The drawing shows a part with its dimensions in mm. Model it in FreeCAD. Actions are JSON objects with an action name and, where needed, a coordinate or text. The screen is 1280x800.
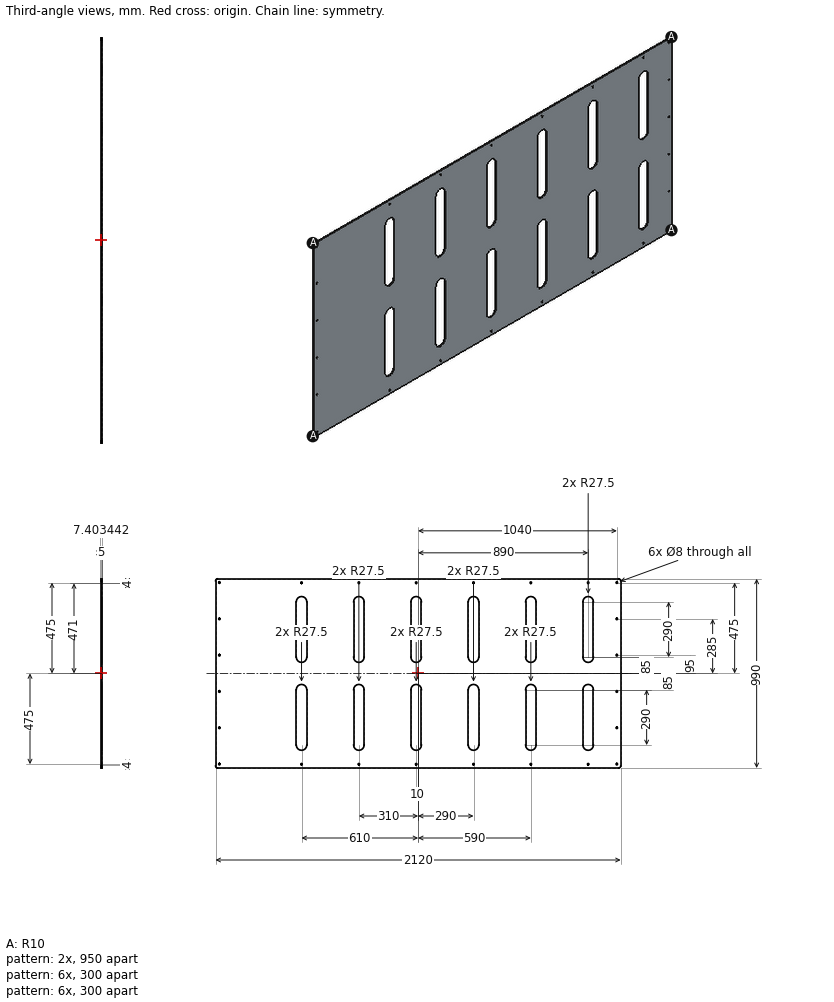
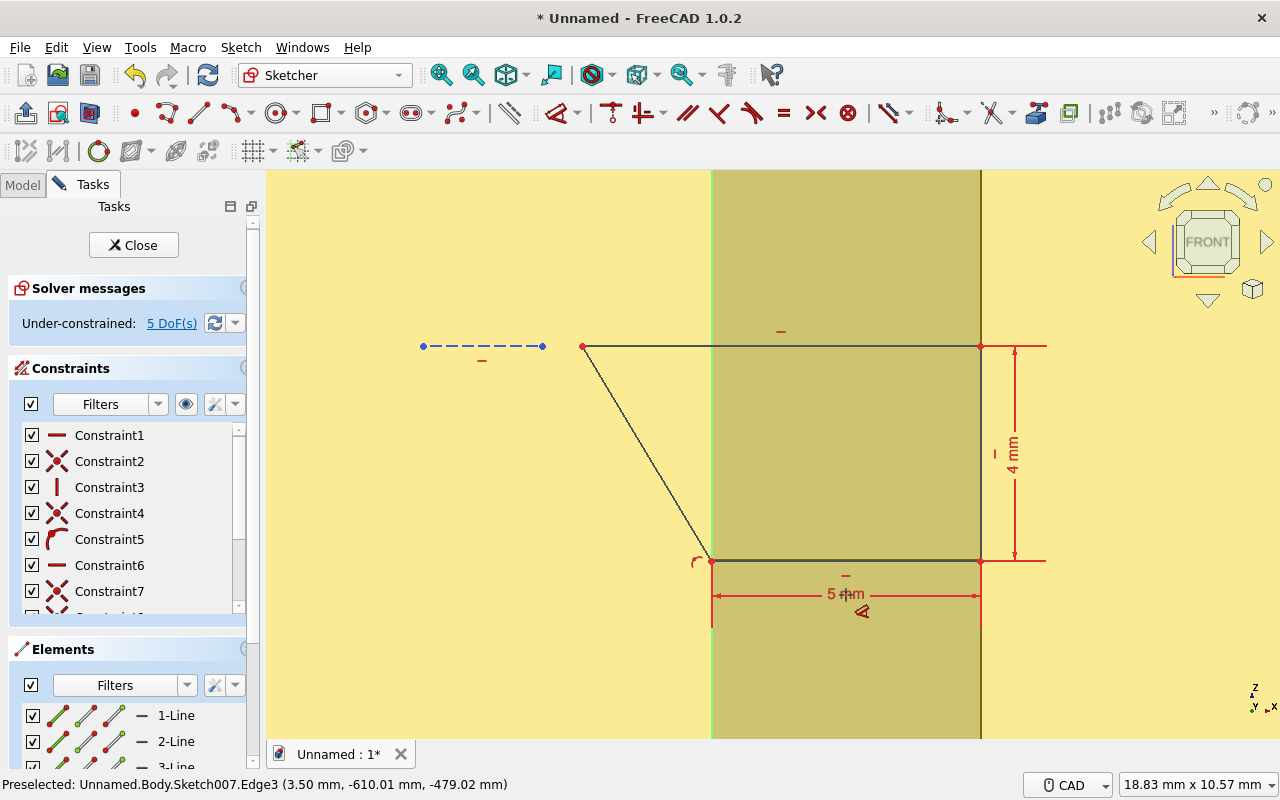
{"action": "left_click", "coordinate": [582, 346]}
{"action": "left_click", "coordinate": [548, 272]}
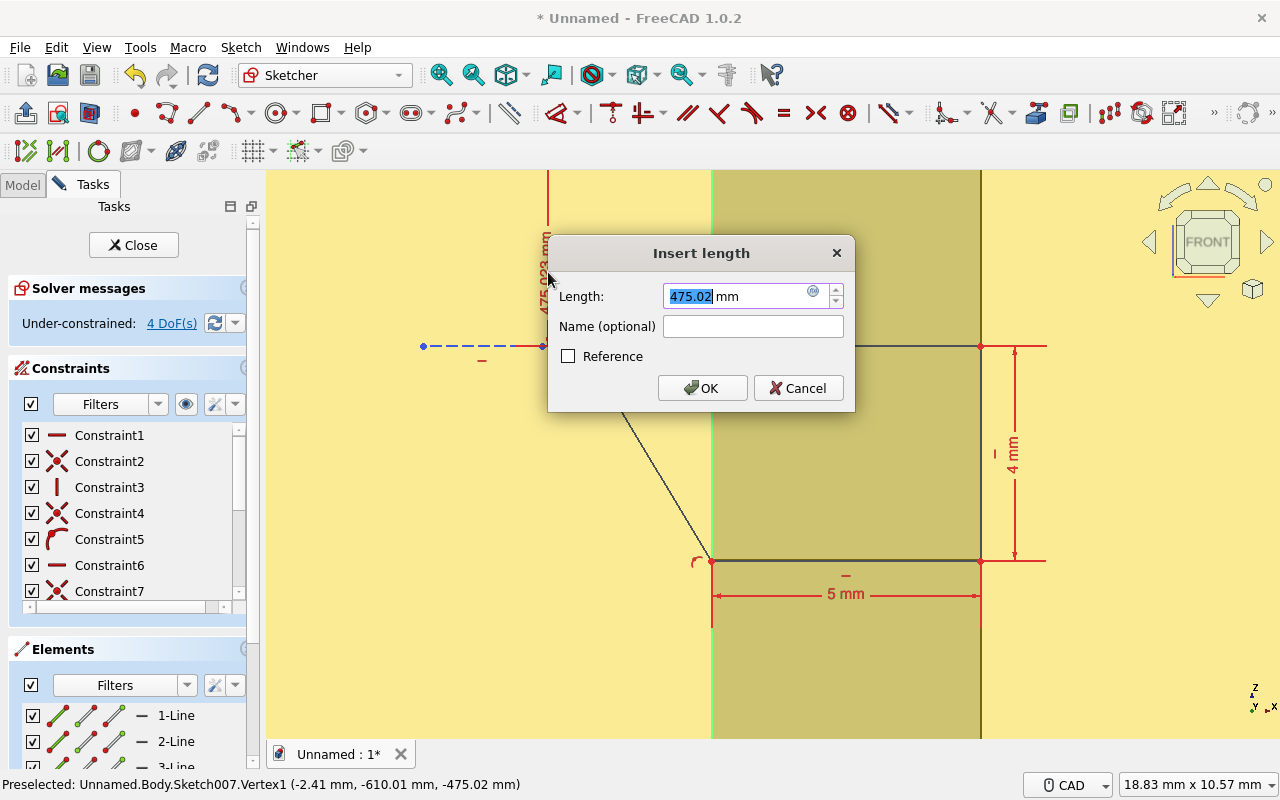
{"action": "type", "text": "475"}
{"action": "key", "text": "Return"}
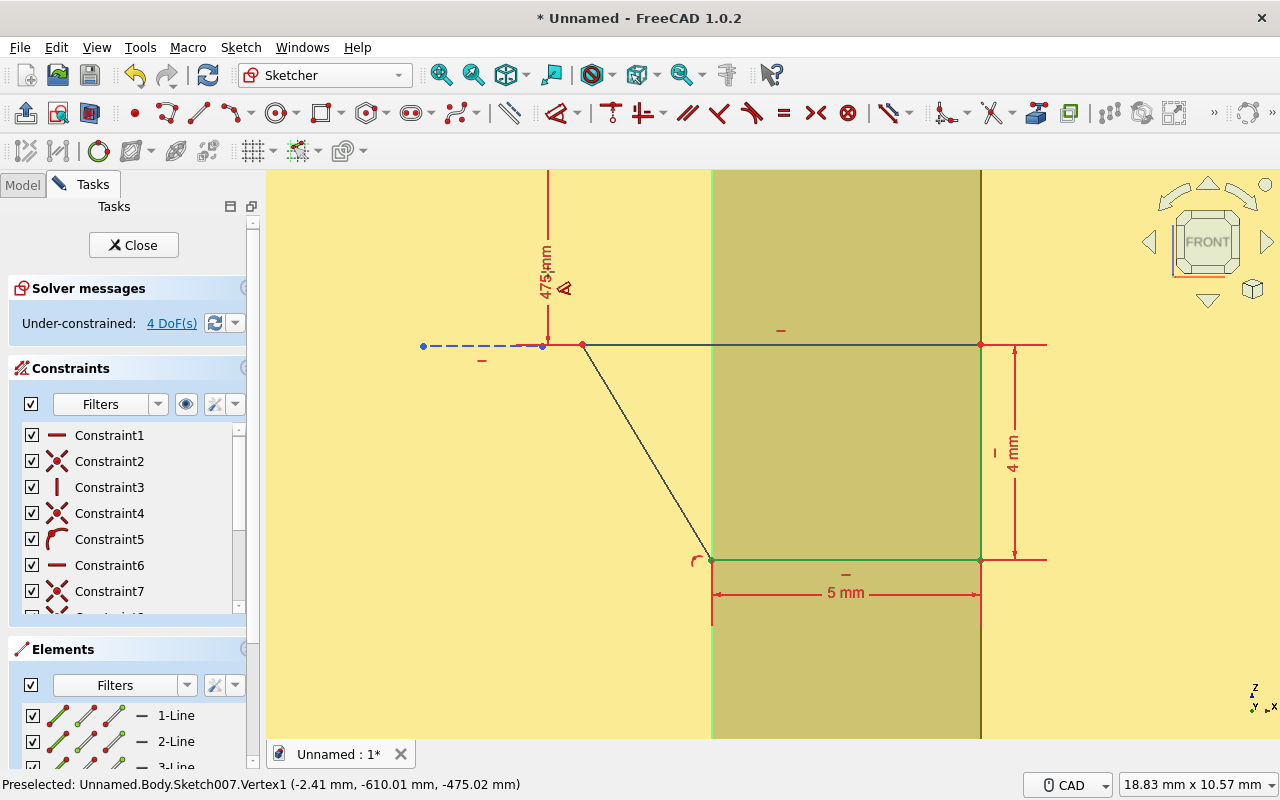
{"action": "left_click", "coordinate": [542, 346]}
{"action": "left_click", "coordinate": [508, 238]}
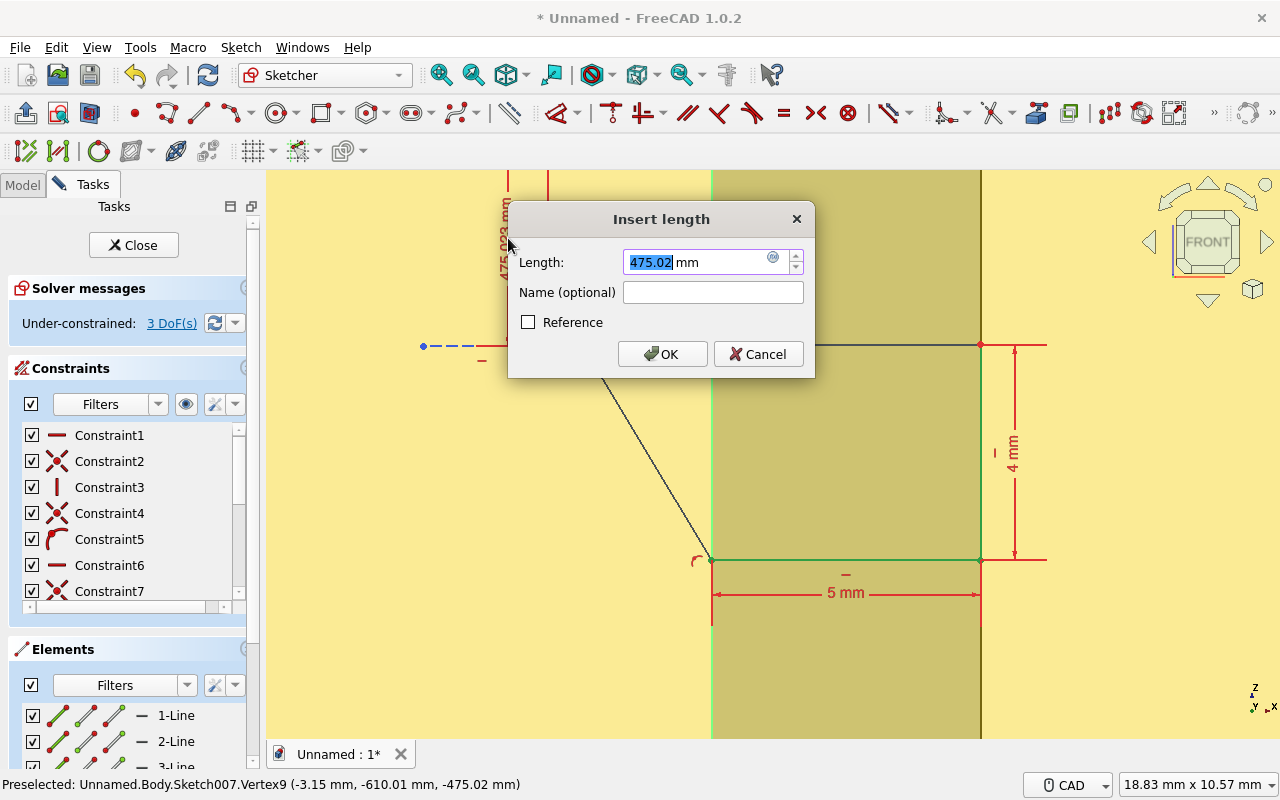
{"action": "type", "text": "475"}
{"action": "key", "text": "Return"}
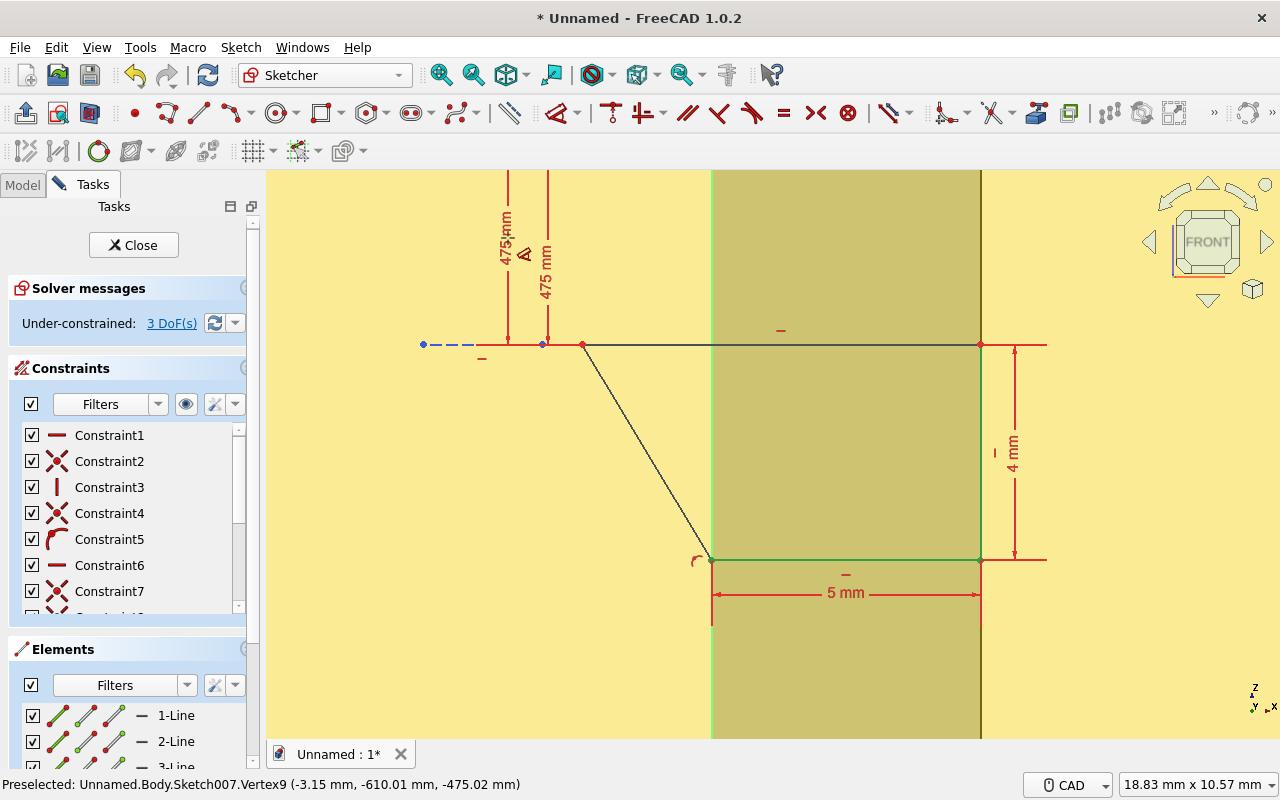
{"action": "scroll", "coordinate": [702, 345], "scroll_direction": "up", "scroll_amount": 2}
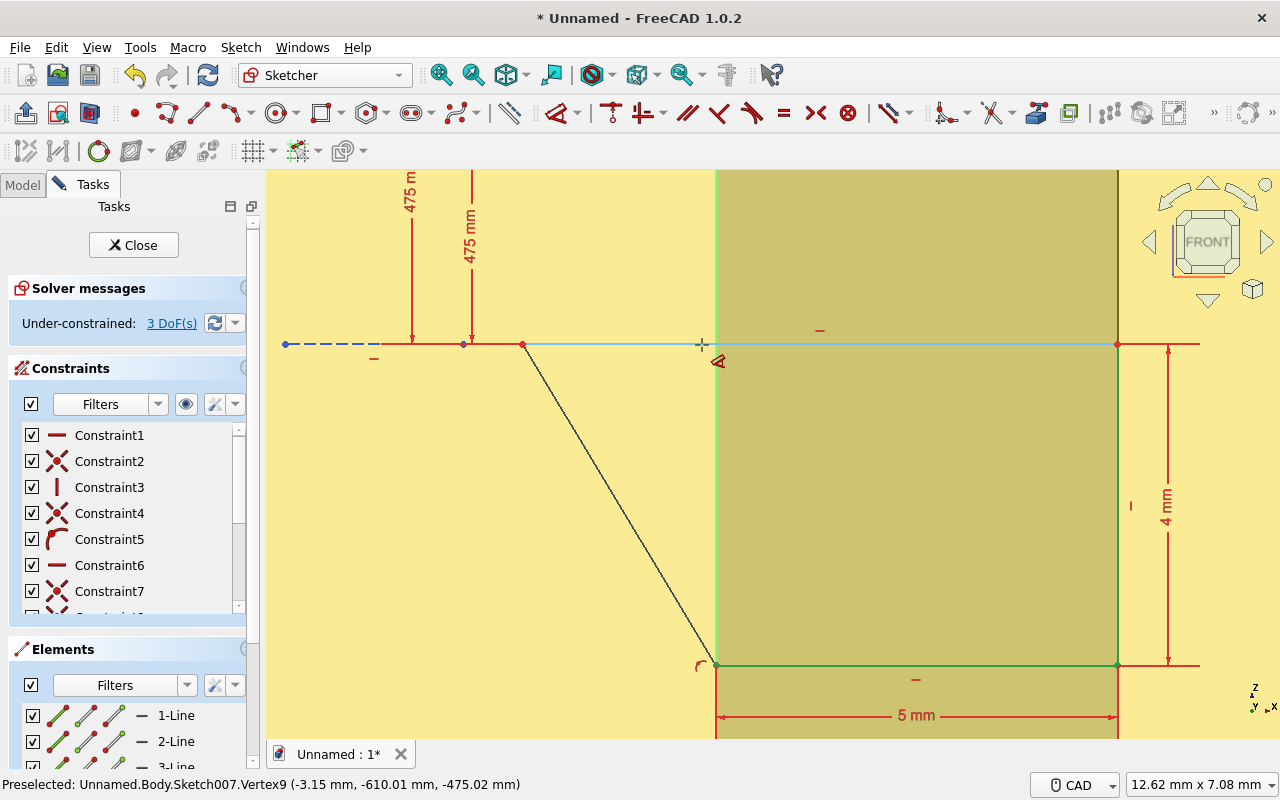
{"action": "left_click", "coordinate": [701, 344]}
{"action": "left_click", "coordinate": [819, 310]}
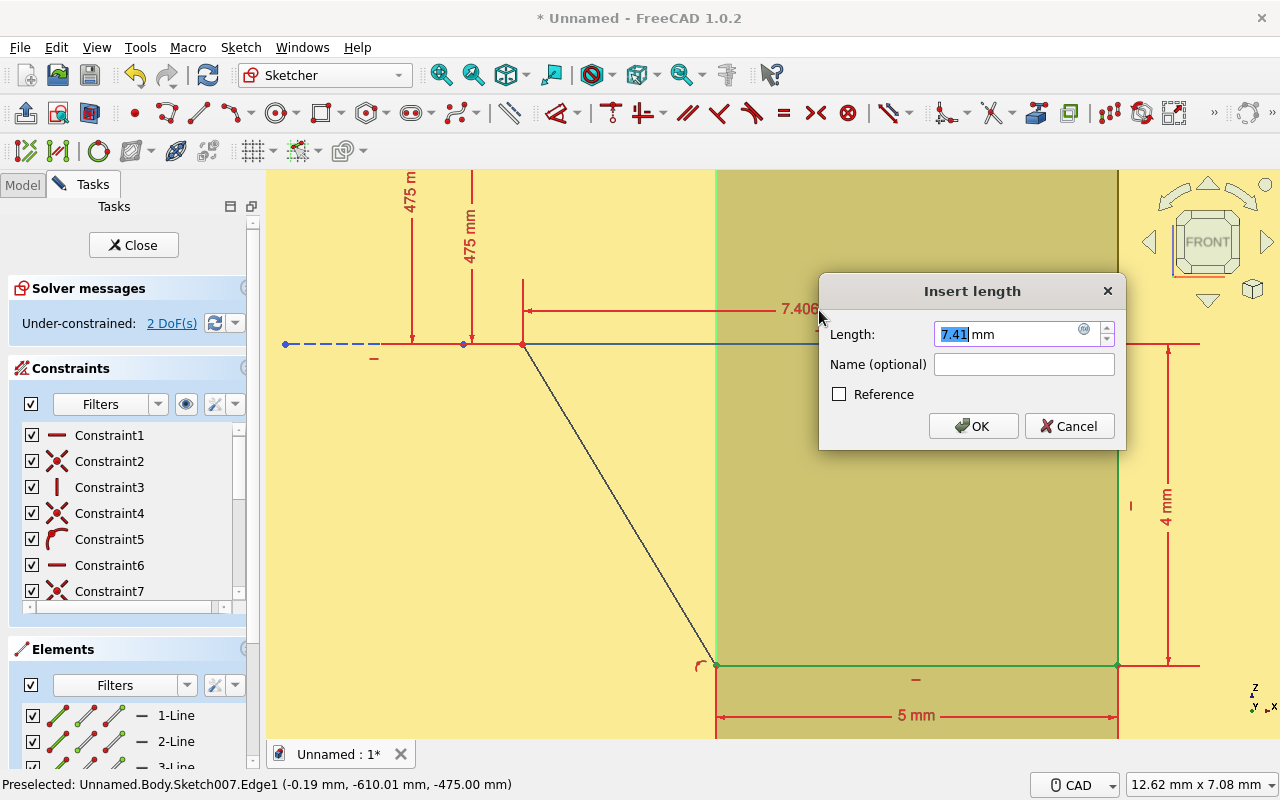
{"action": "type", "text": "7.403442"}
{"action": "key", "text": "Return"}
{"action": "key", "text": "Escape"}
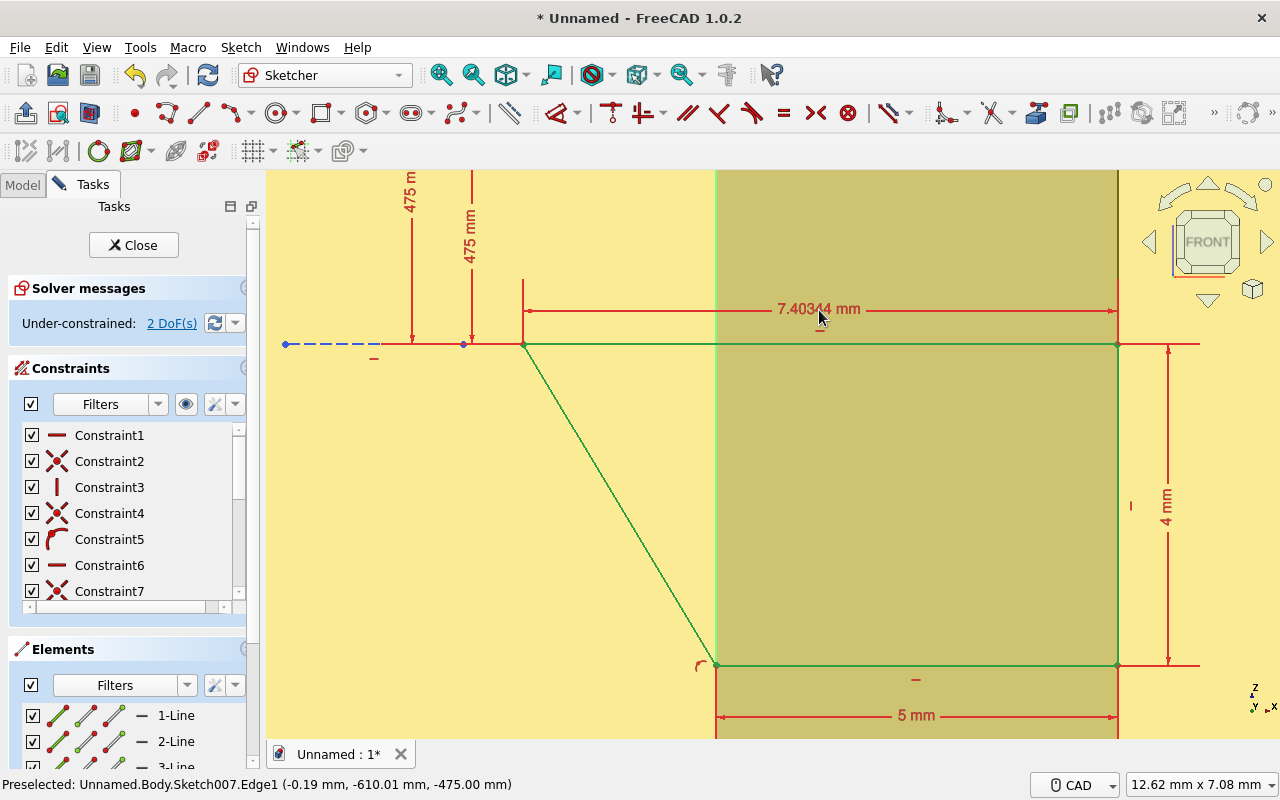
{"action": "left_click", "coordinate": [134, 245]}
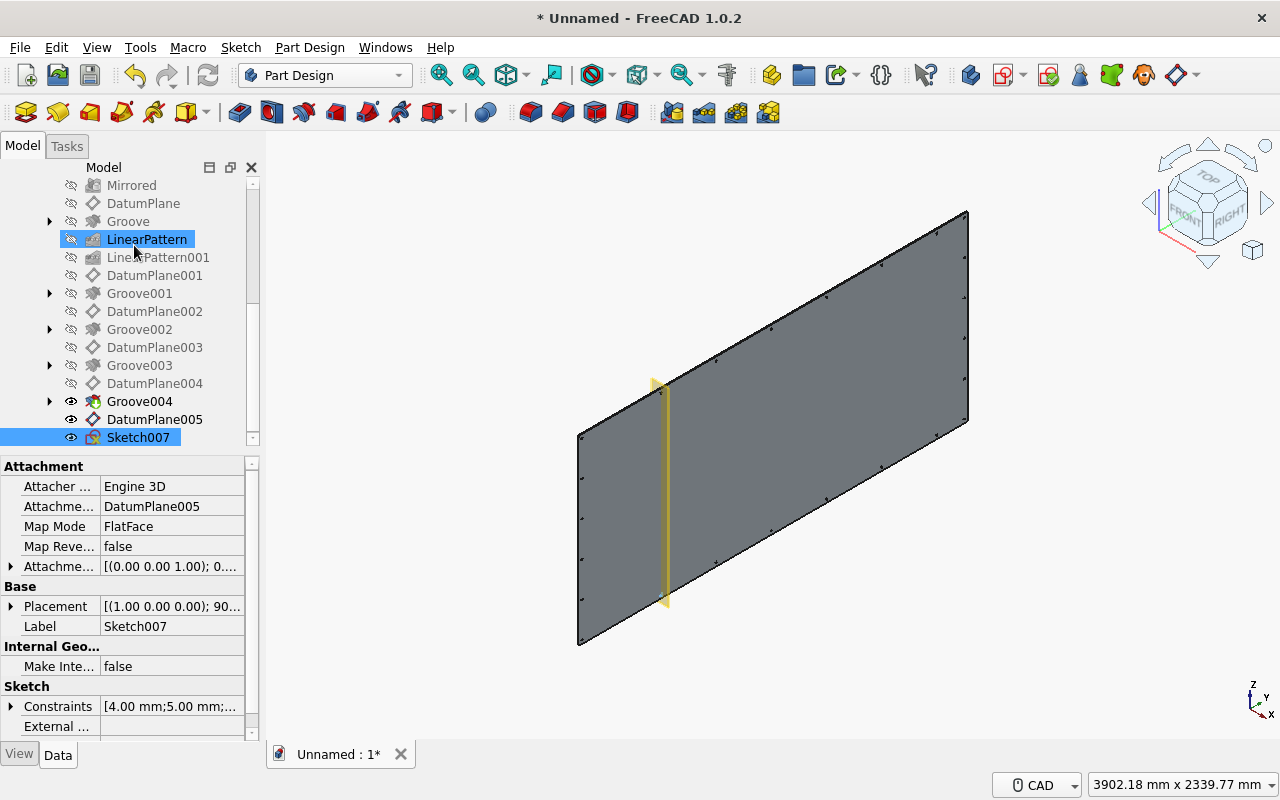
{"action": "left_click", "coordinate": [304, 112]}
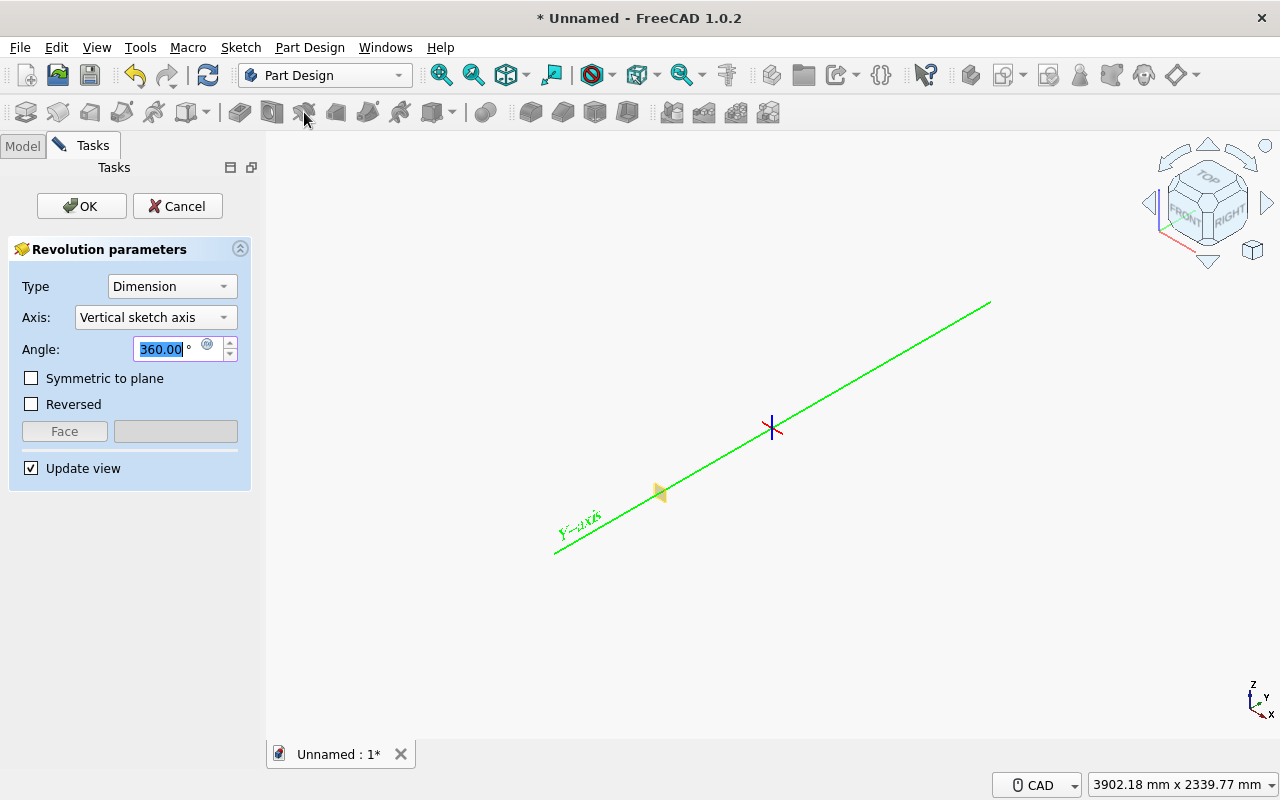
{"action": "left_click", "coordinate": [156, 318]}